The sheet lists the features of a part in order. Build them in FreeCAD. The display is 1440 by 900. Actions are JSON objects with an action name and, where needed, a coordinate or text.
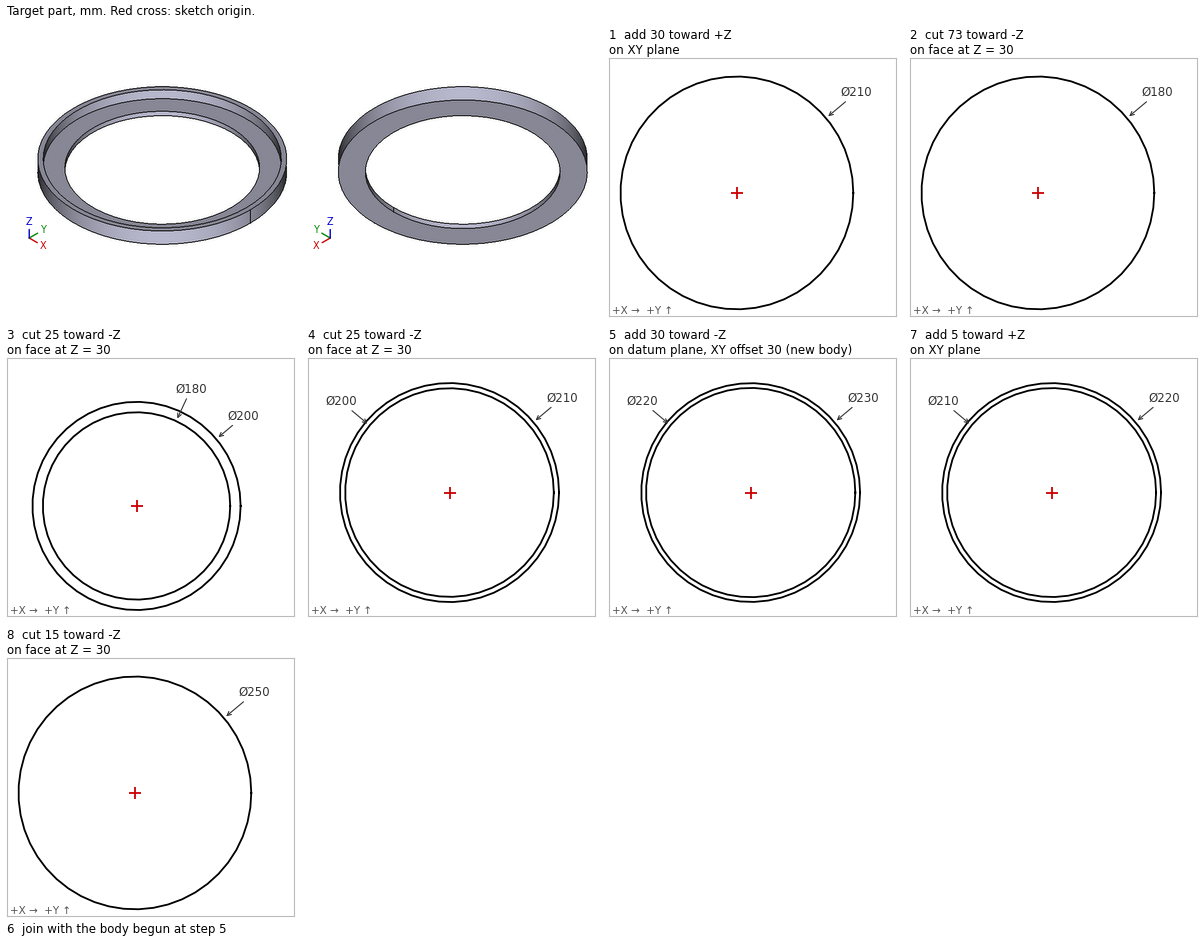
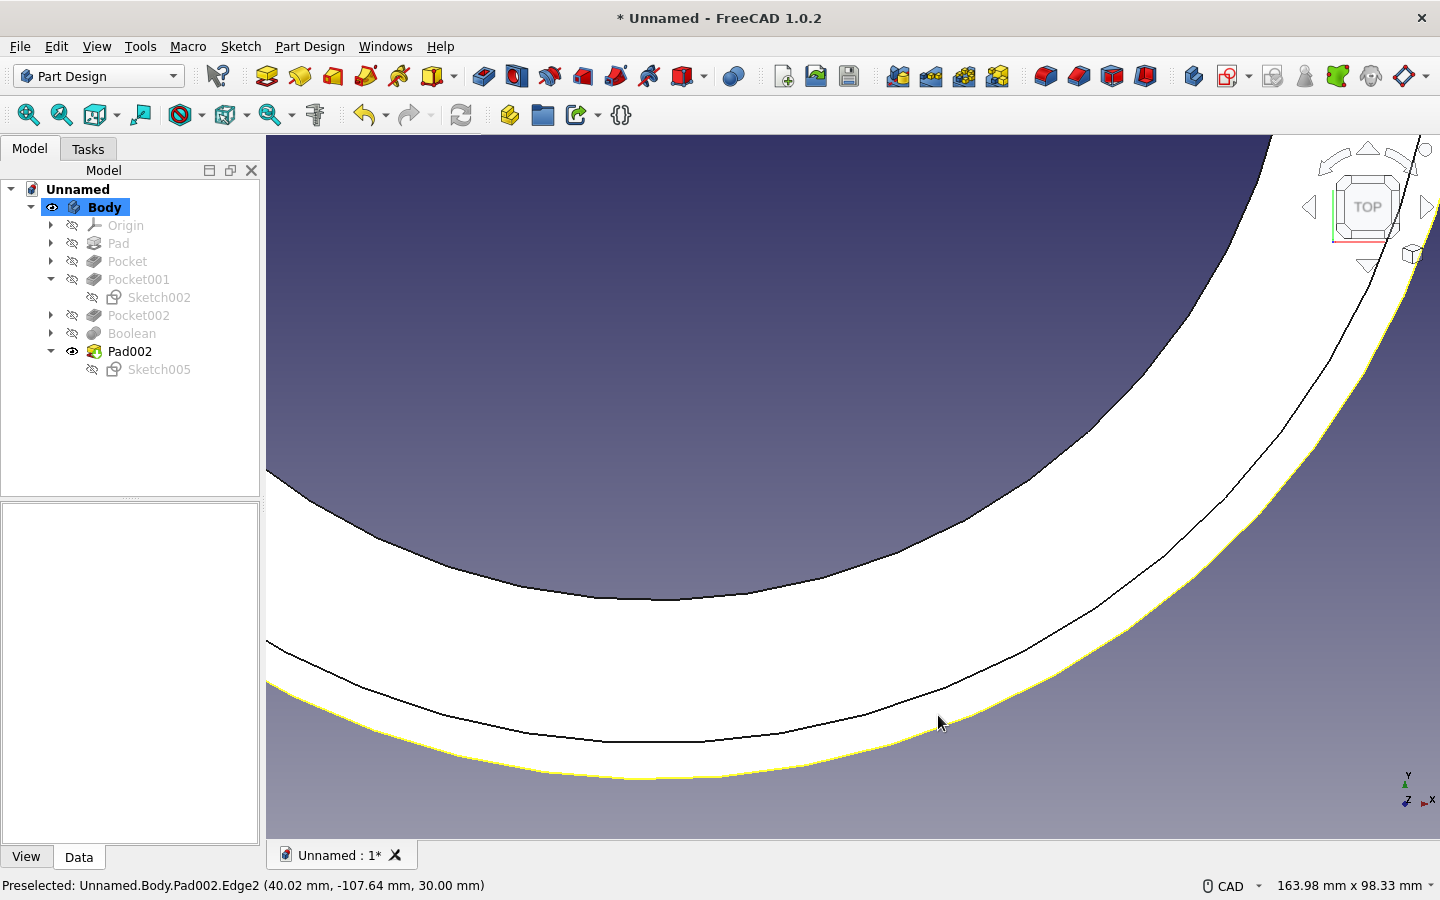
{"action": "left_click", "coordinate": [937, 715]}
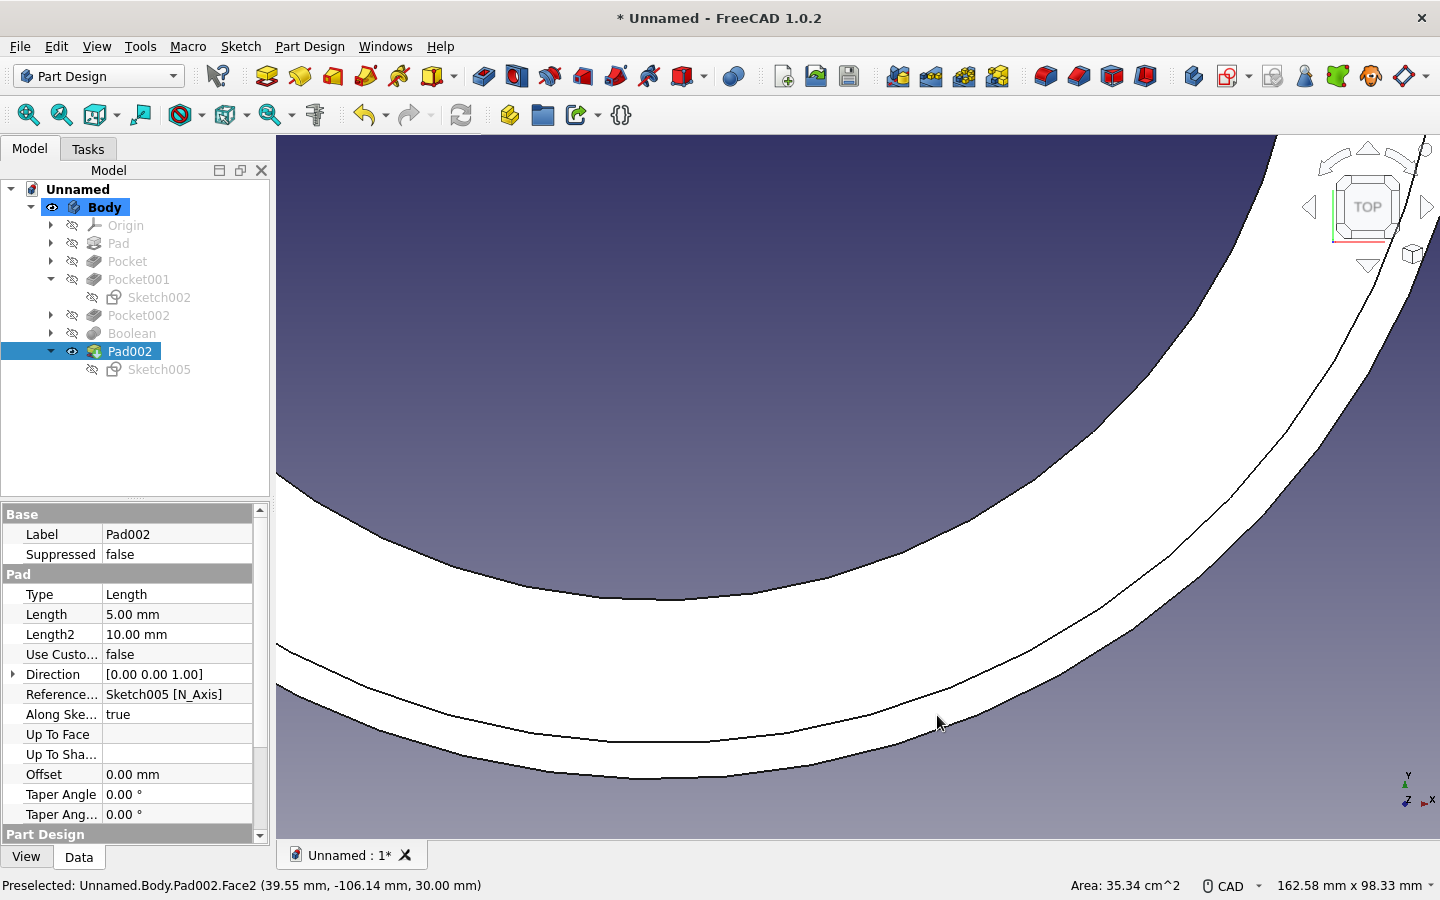
{"action": "left_click", "coordinate": [1226, 76]}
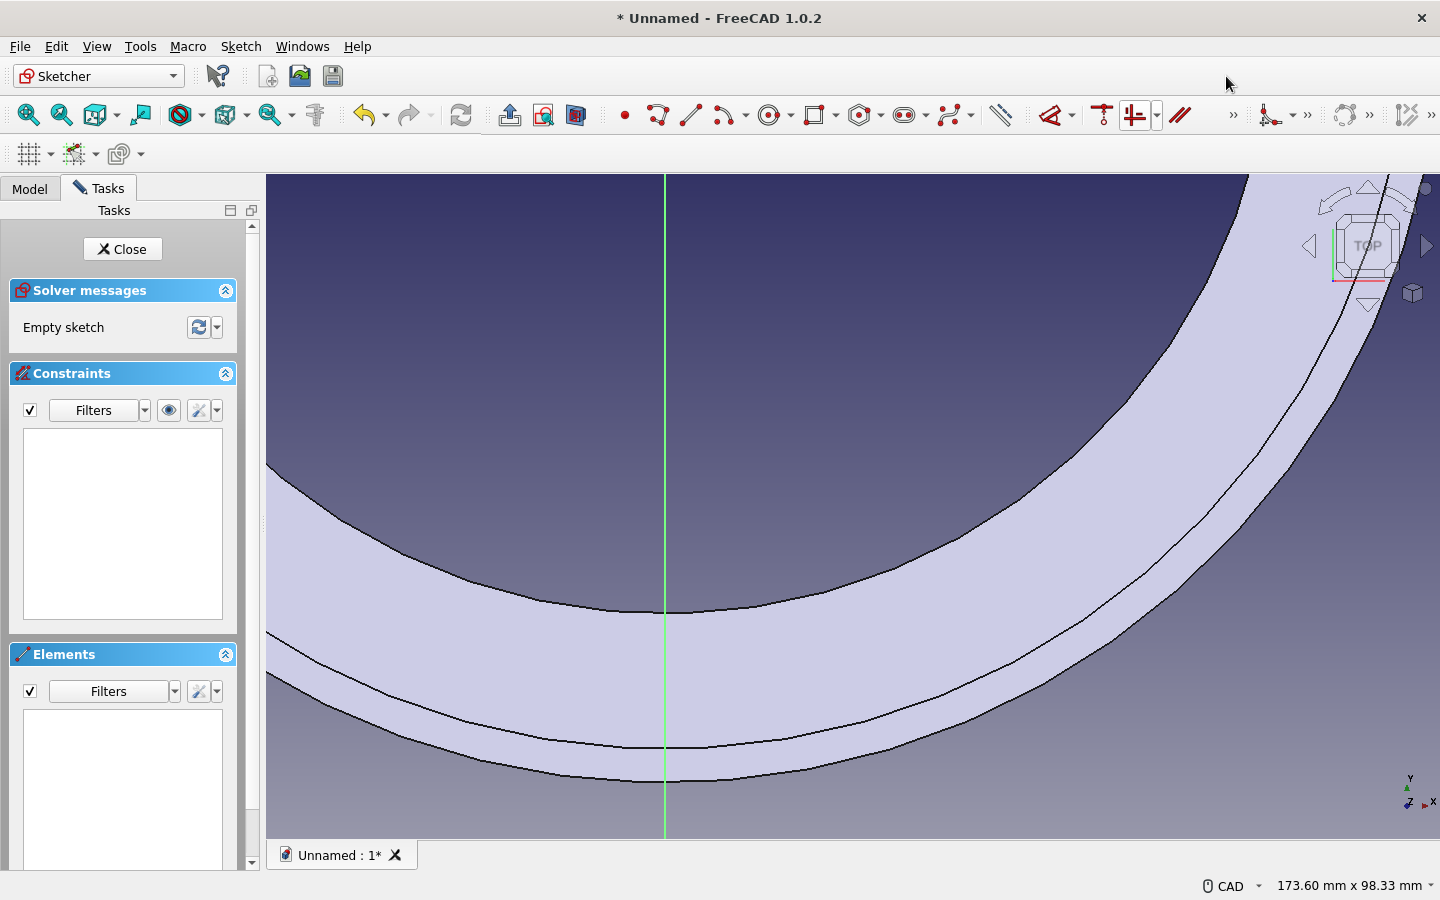
{"action": "scroll", "coordinate": [824, 671], "scroll_direction": "down", "scroll_amount": 7}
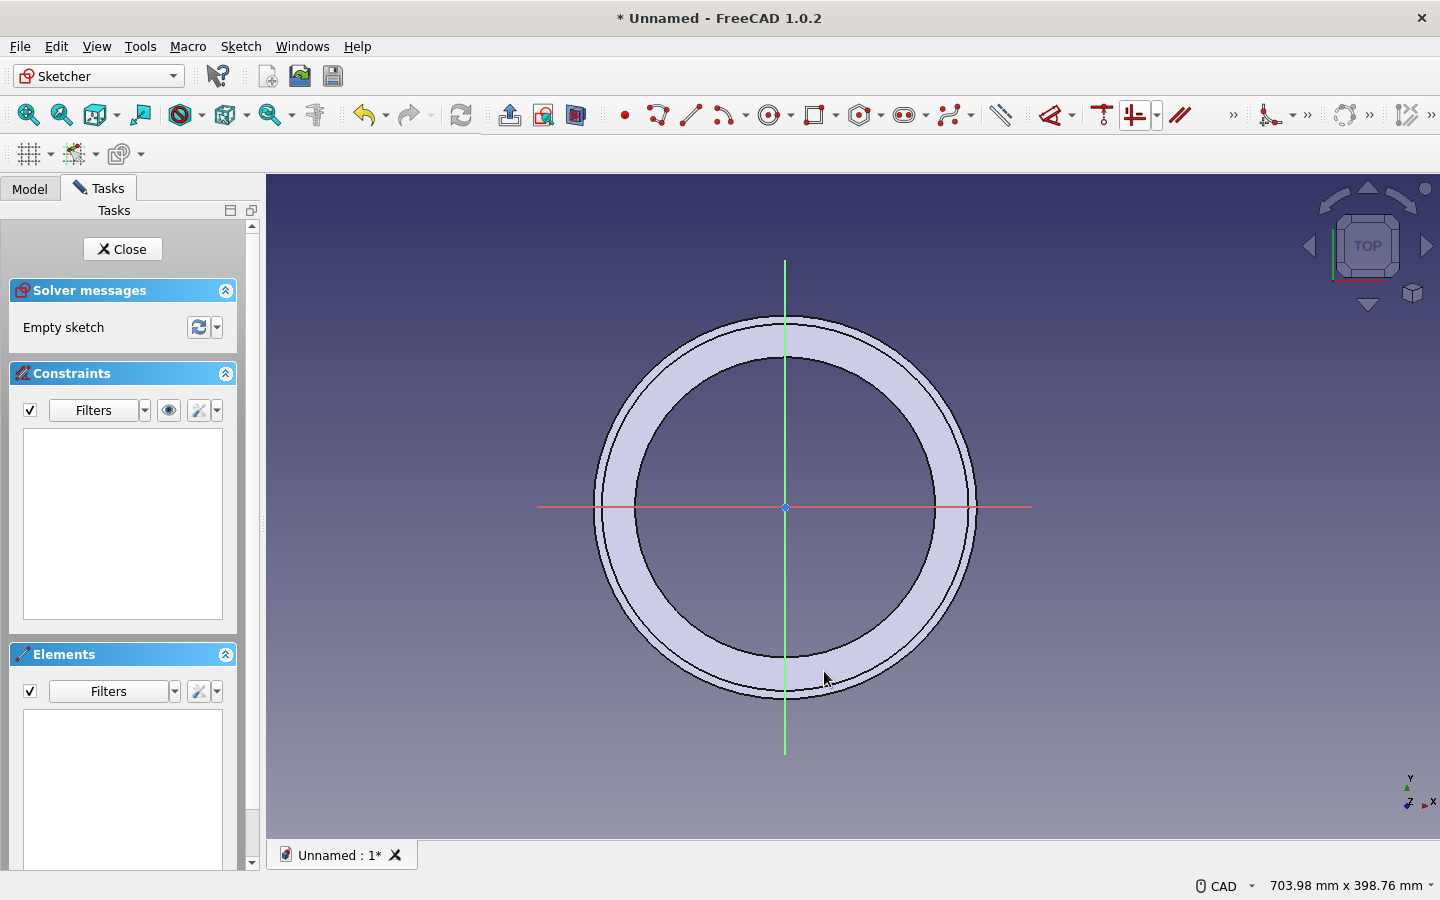
{"action": "left_click", "coordinate": [768, 116]}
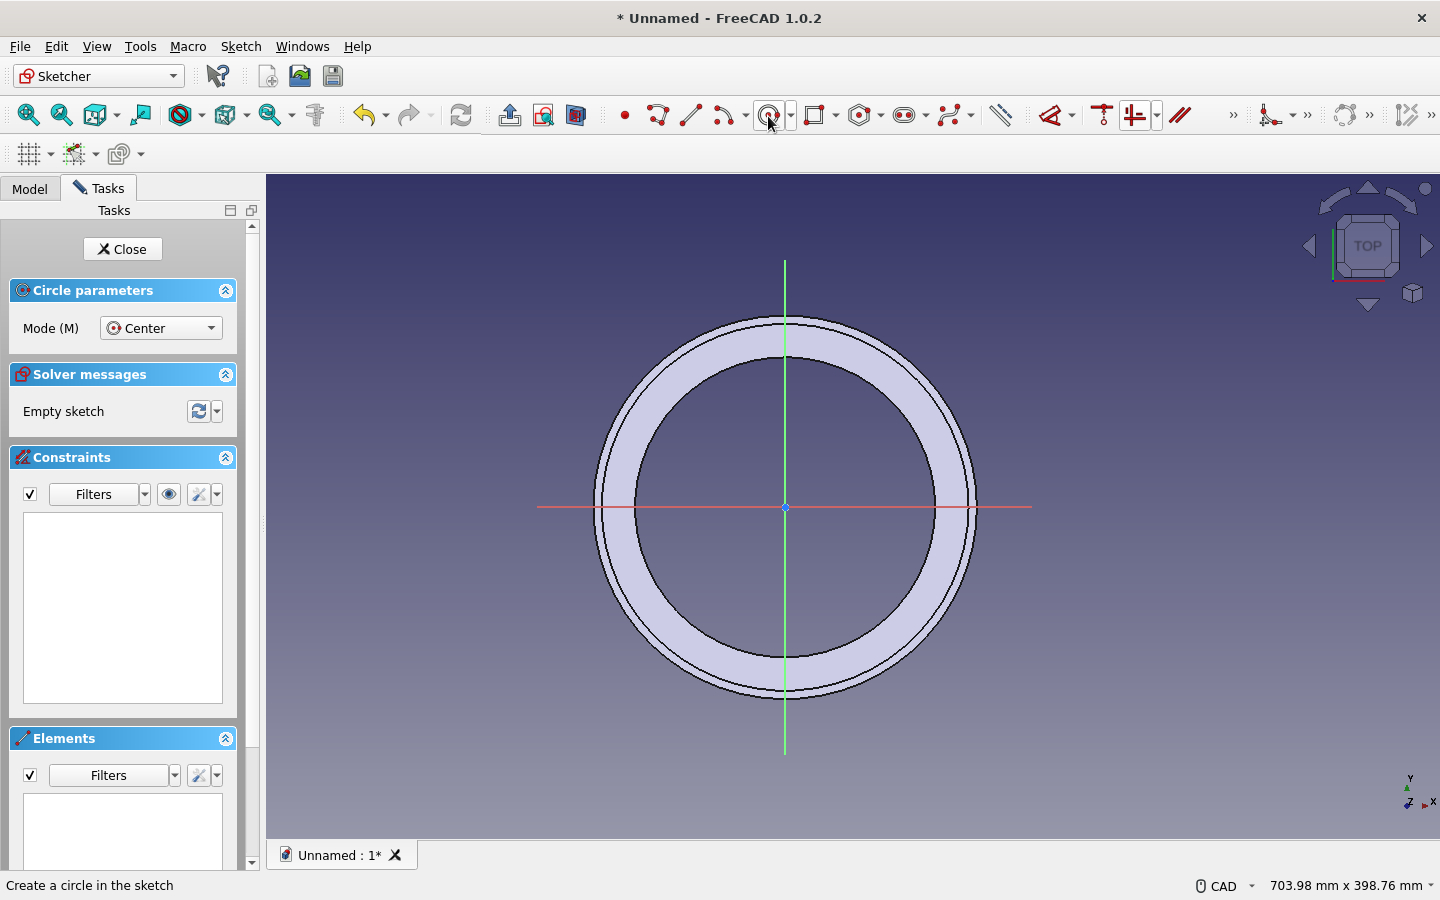
{"action": "left_click", "coordinate": [785, 507]}
{"action": "mouse_move", "coordinate": [933, 360]}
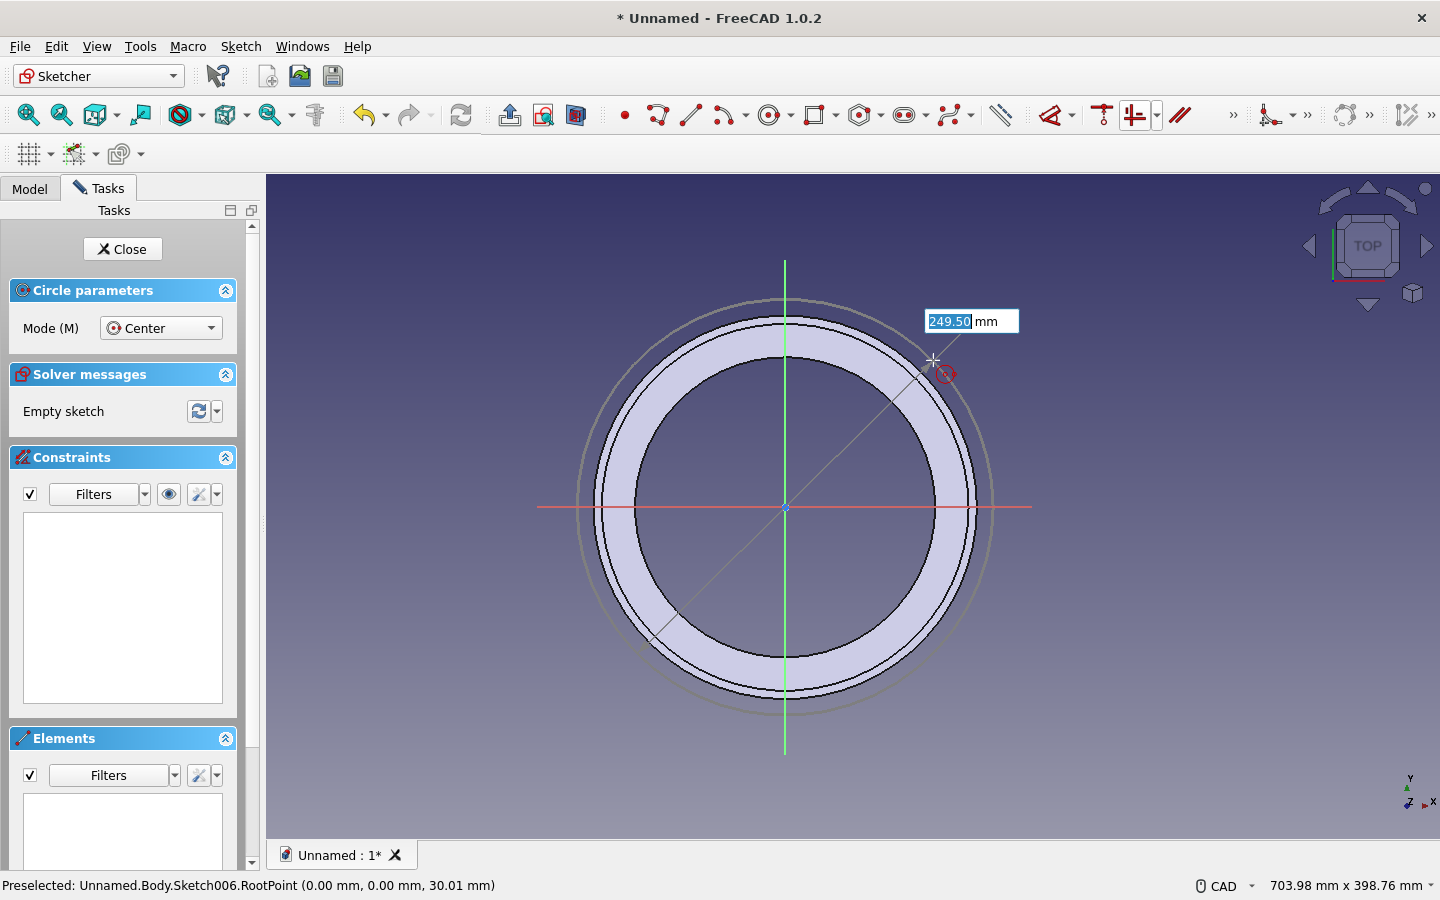
{"action": "type", "text": "250"}
{"action": "key", "text": "Return"}
{"action": "key", "text": "Escape"}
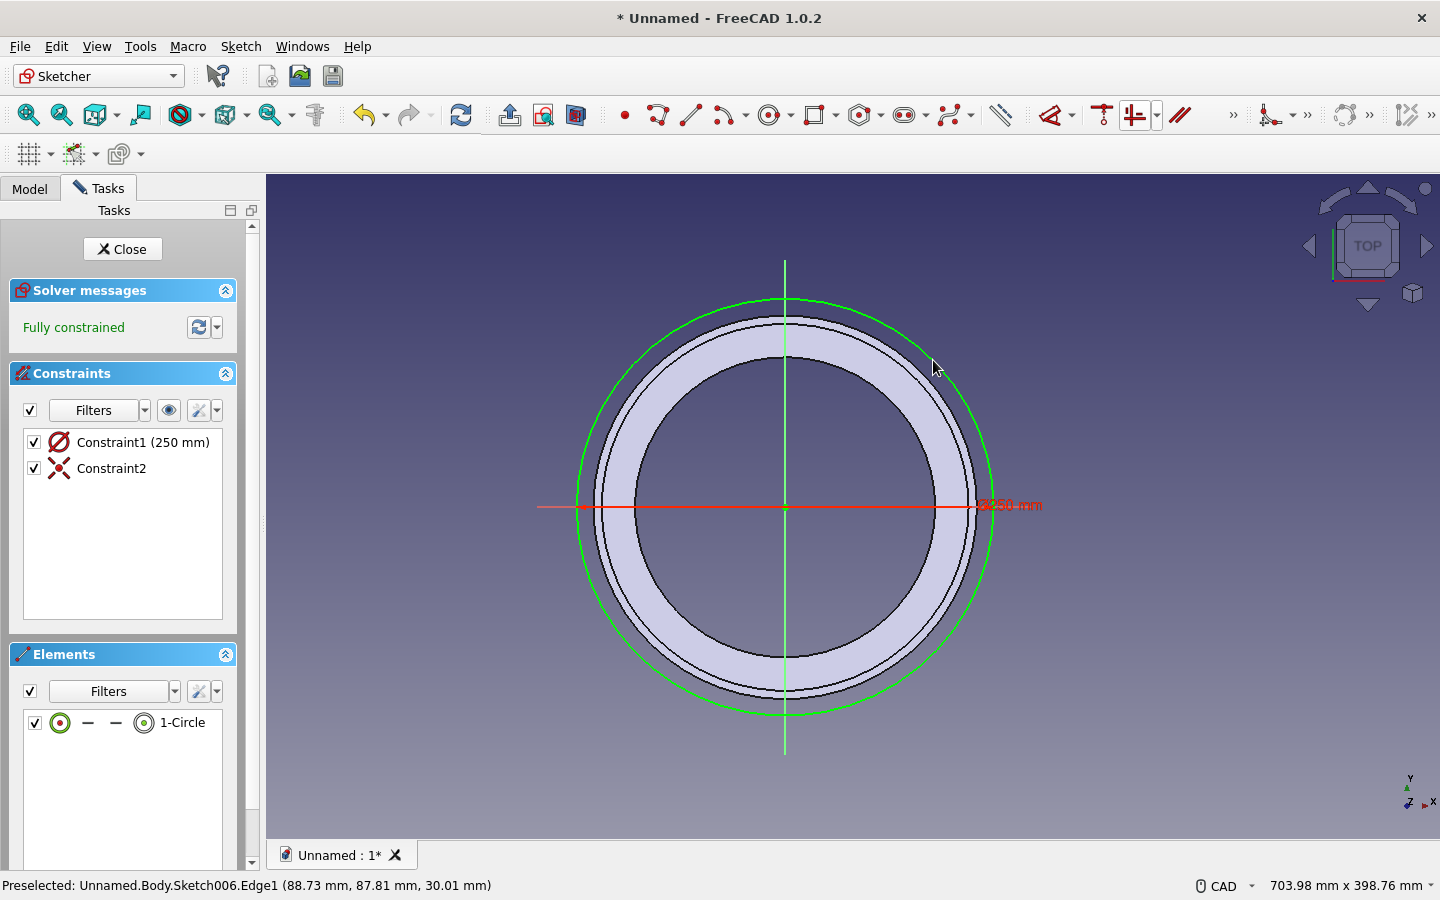
{"action": "left_click", "coordinate": [123, 249]}